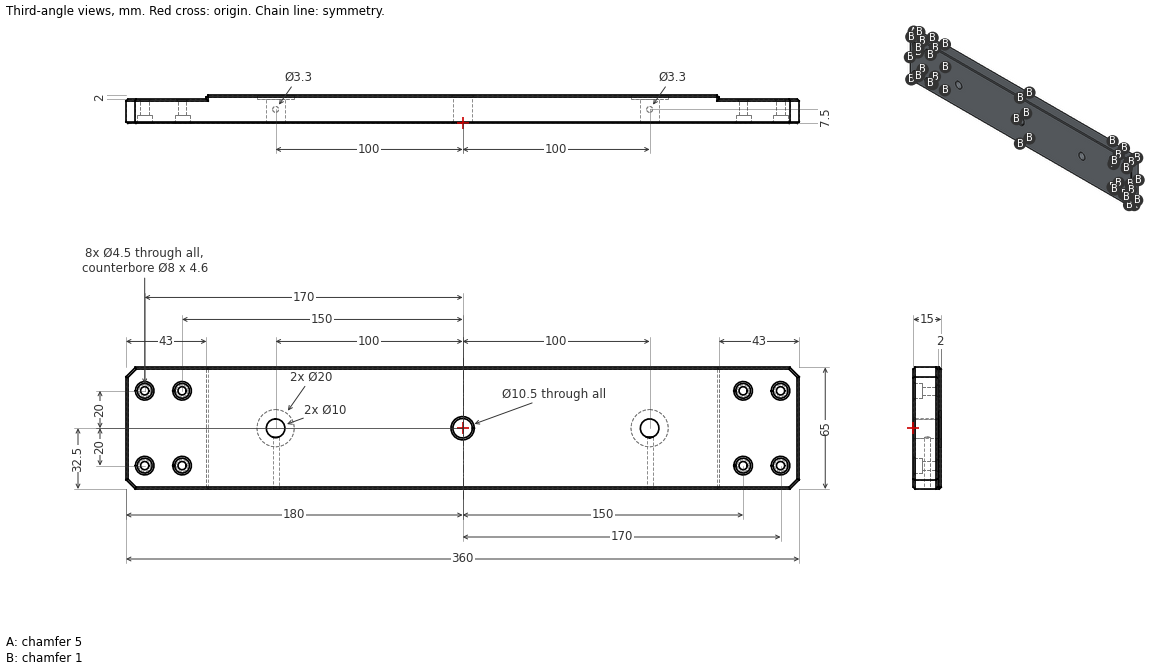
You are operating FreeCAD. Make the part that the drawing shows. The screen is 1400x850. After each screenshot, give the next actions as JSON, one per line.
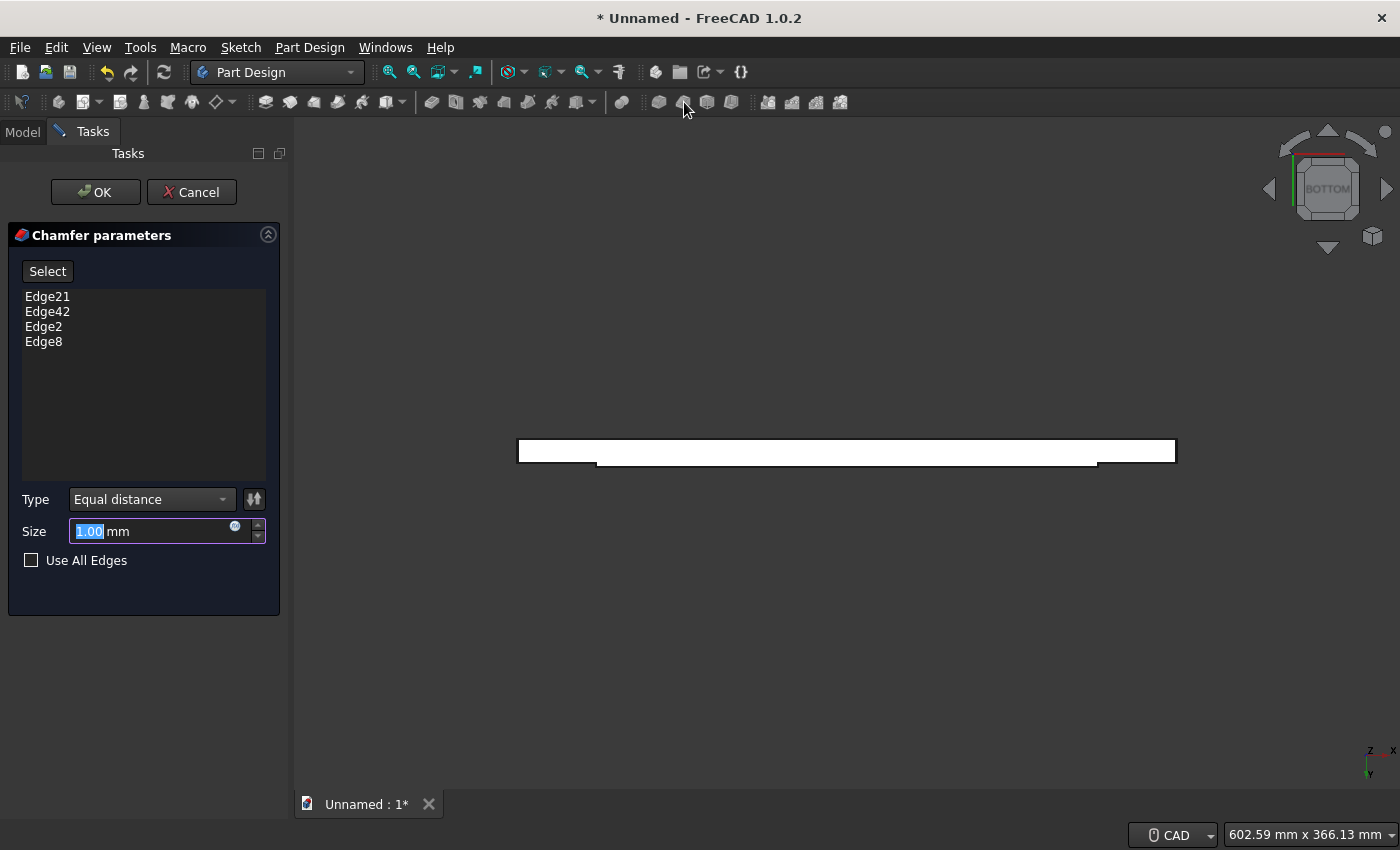
{"action": "type", "text": "5"}
{"action": "key", "text": "Tab"}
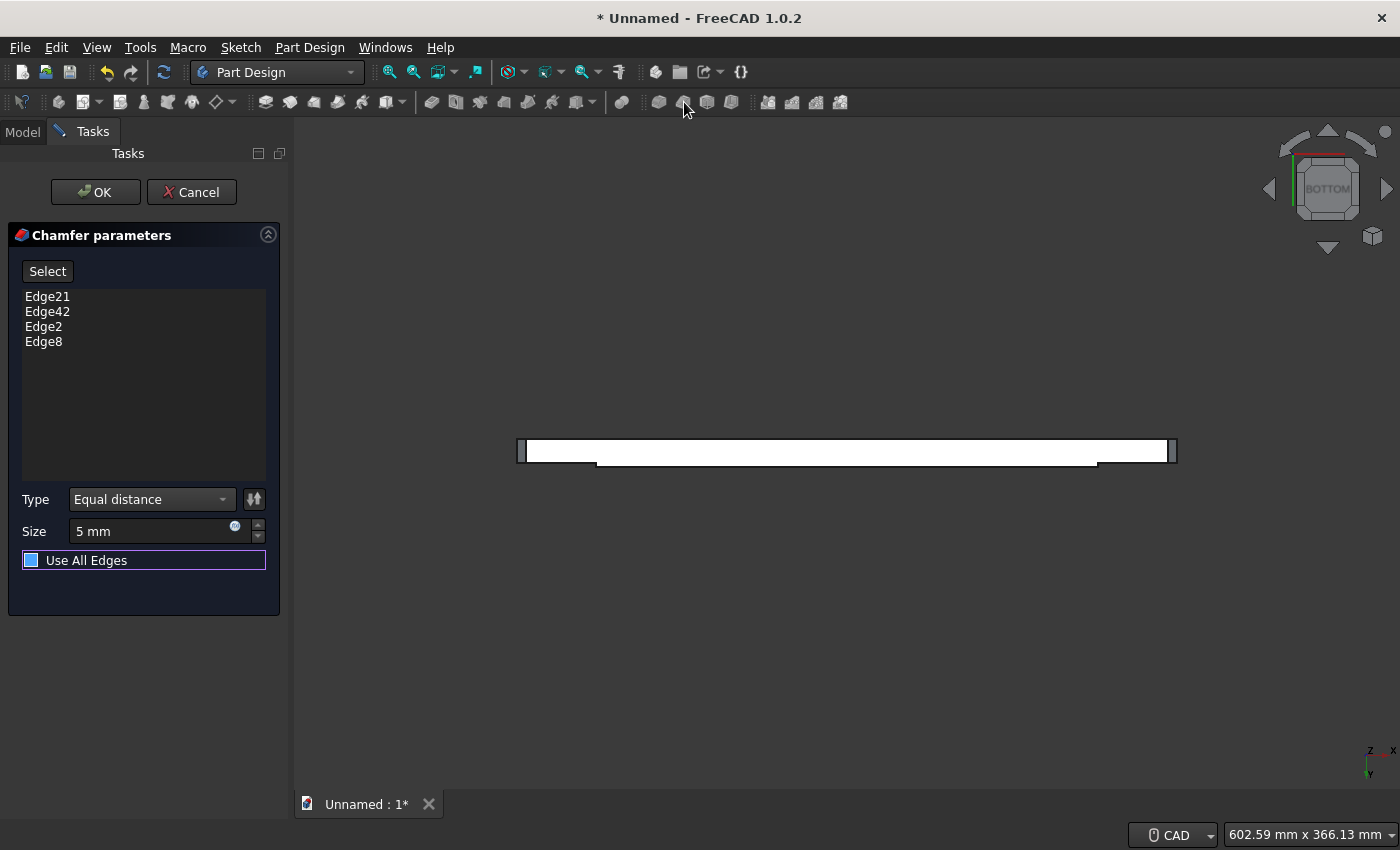
{"action": "left_click", "coordinate": [96, 192]}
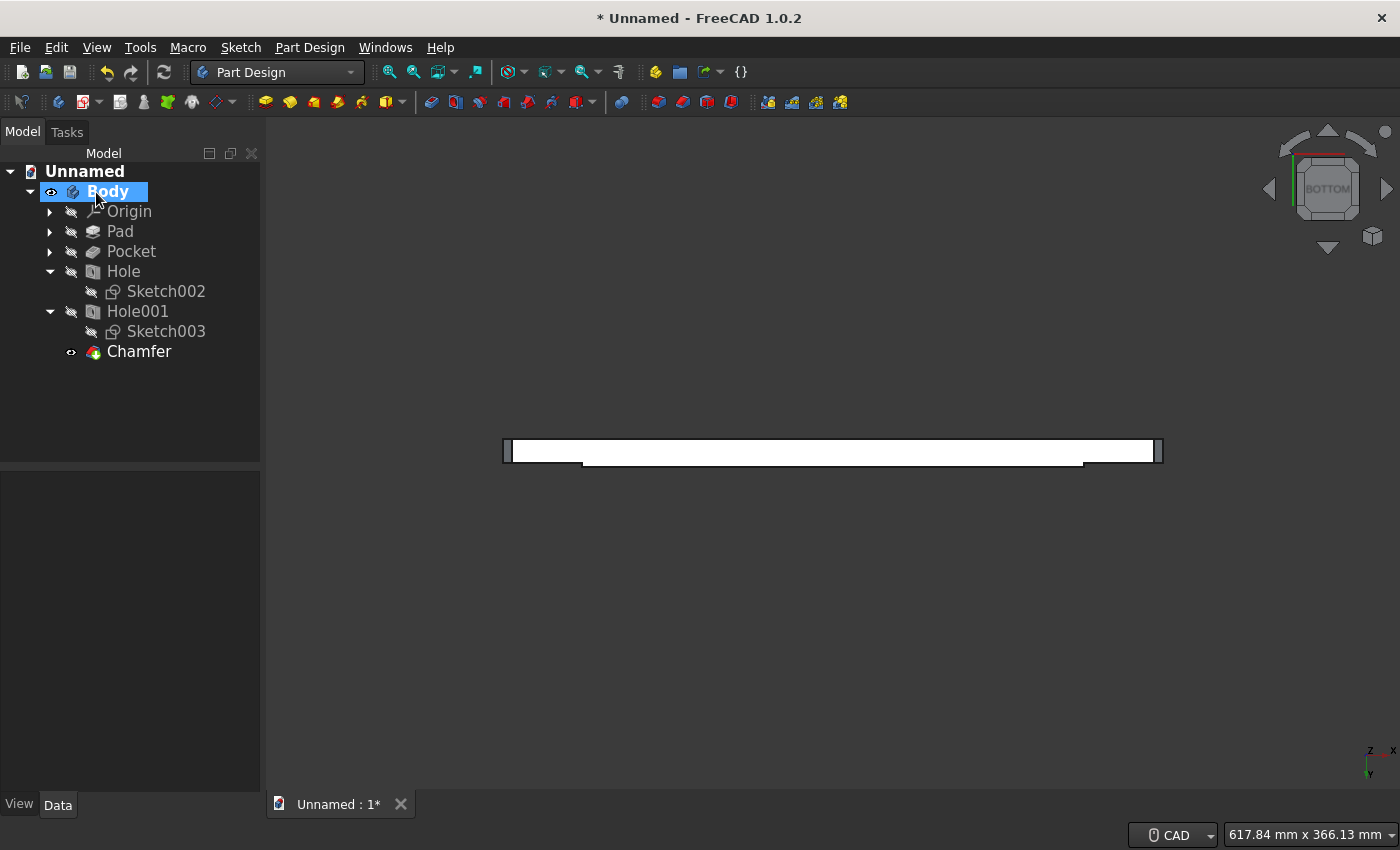
{"action": "key", "text": "0"}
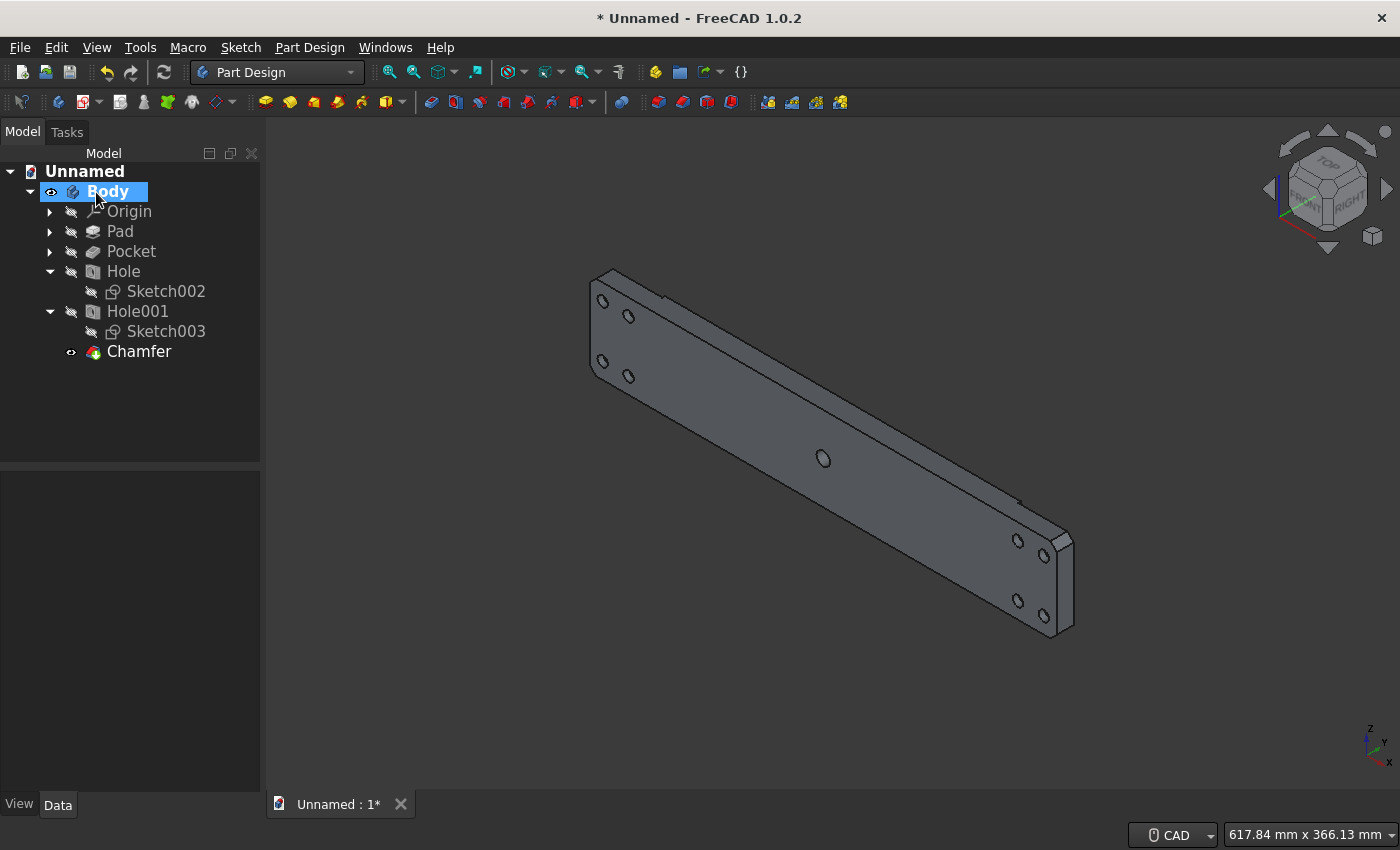
{"action": "left_click", "coordinate": [957, 535]}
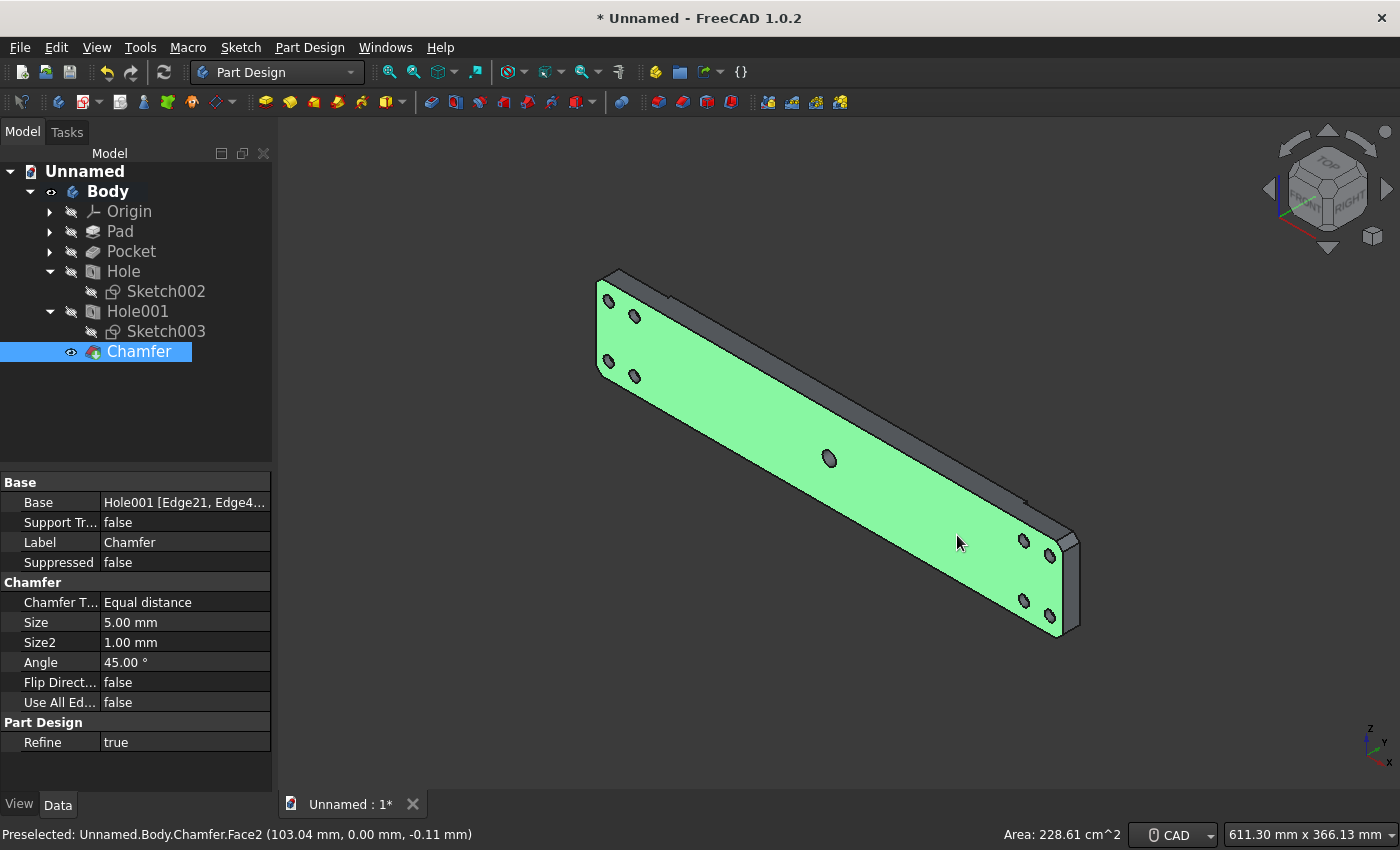
{"action": "key", "text": "2"}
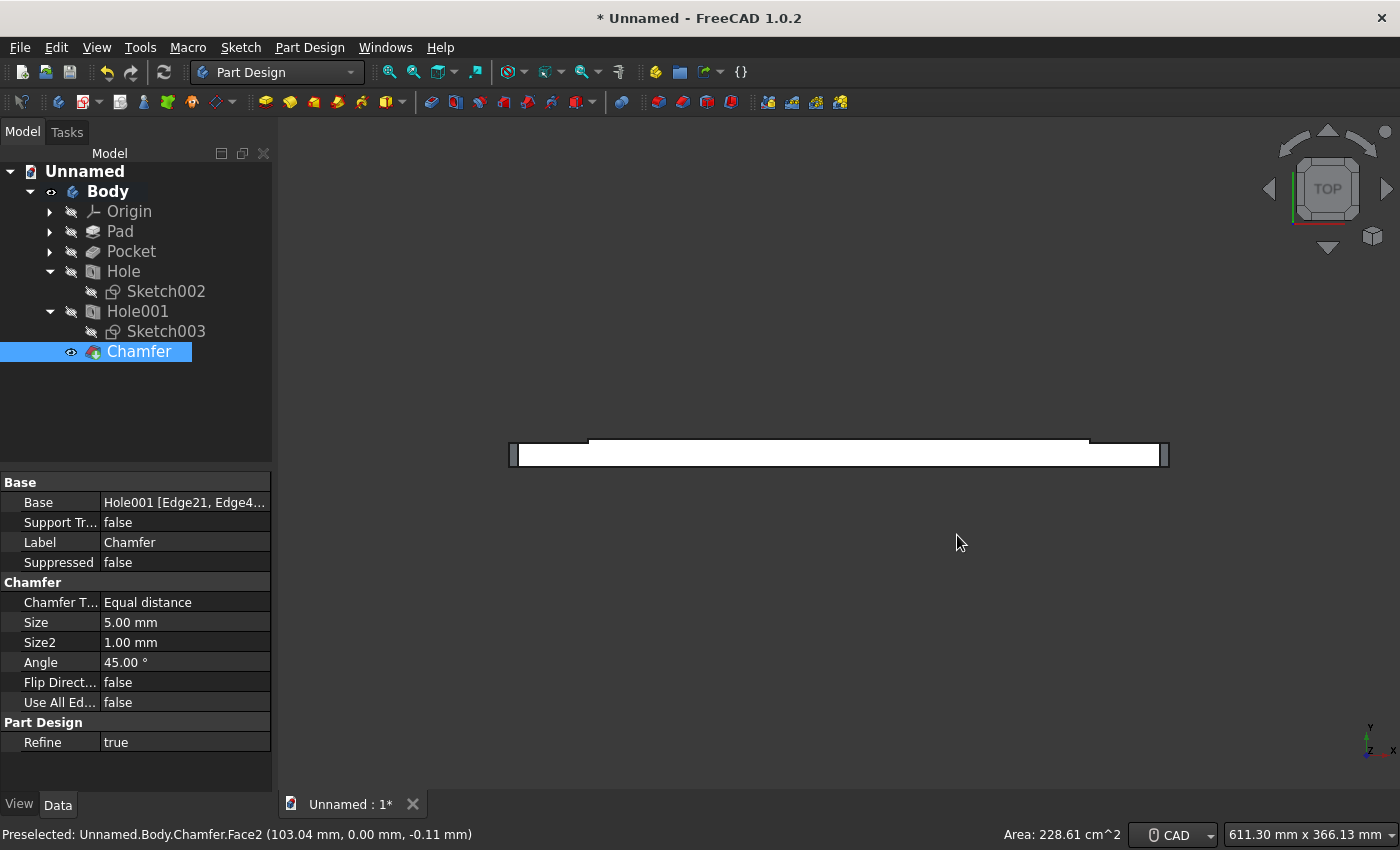
{"action": "left_click", "coordinate": [553, 442], "text": "ctrl"}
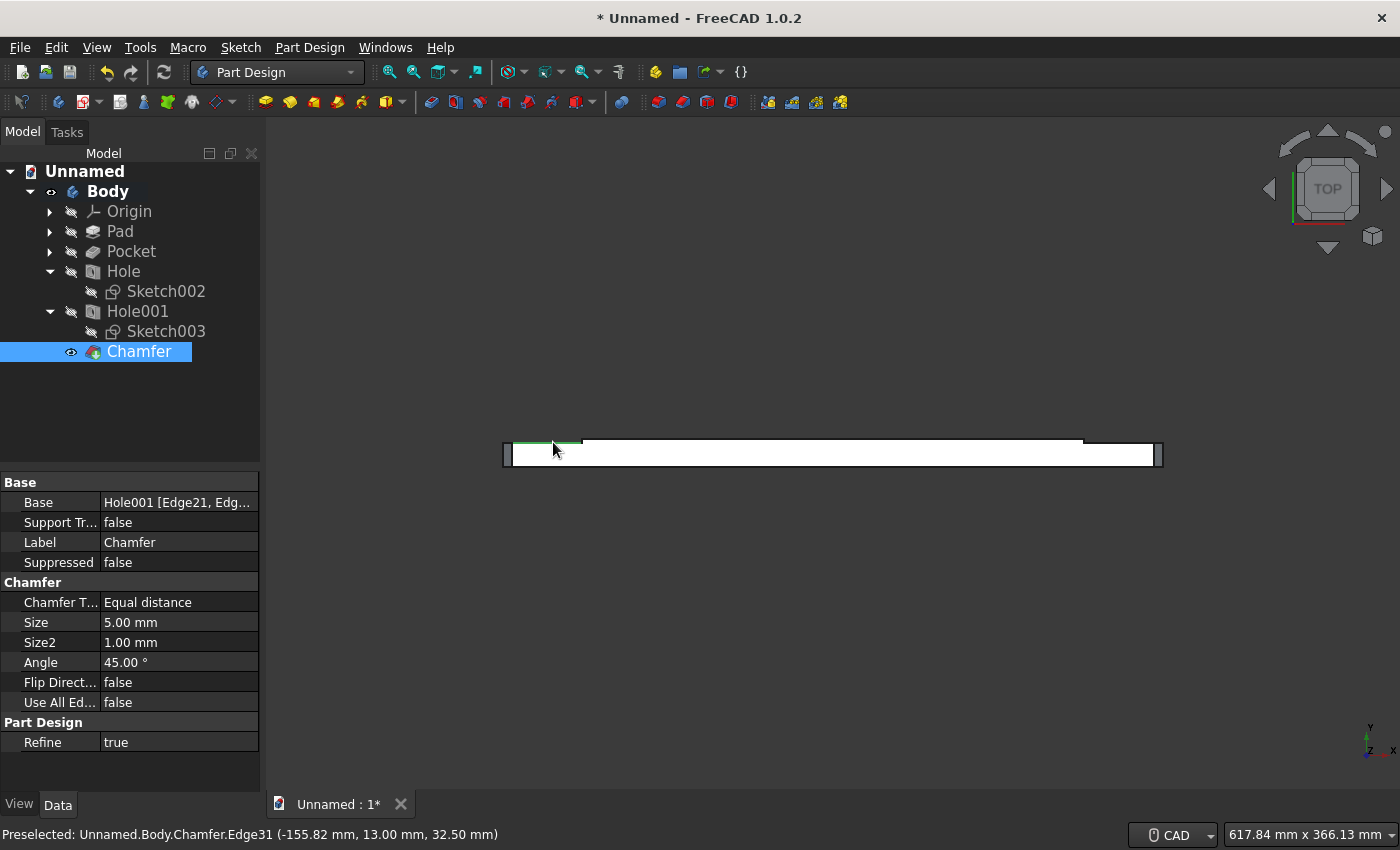
{"action": "left_click", "coordinate": [505, 442], "text": "ctrl"}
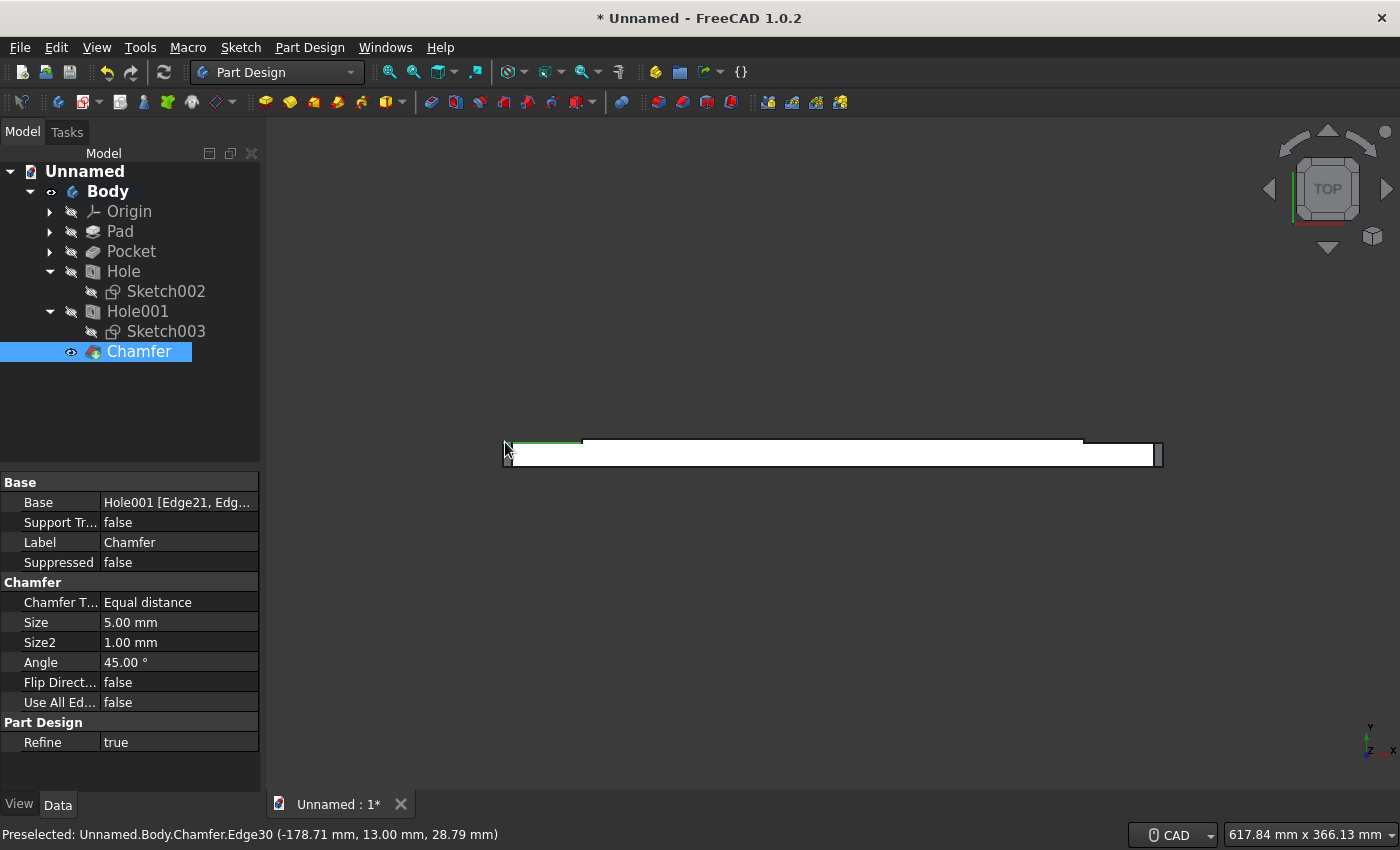
{"action": "left_click", "coordinate": [1161, 442], "text": "ctrl"}